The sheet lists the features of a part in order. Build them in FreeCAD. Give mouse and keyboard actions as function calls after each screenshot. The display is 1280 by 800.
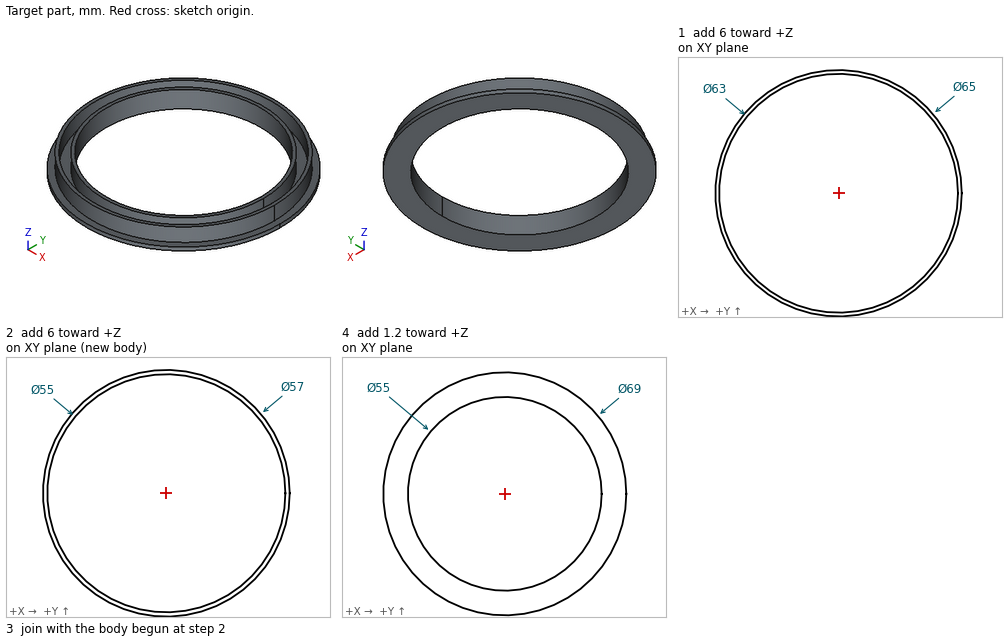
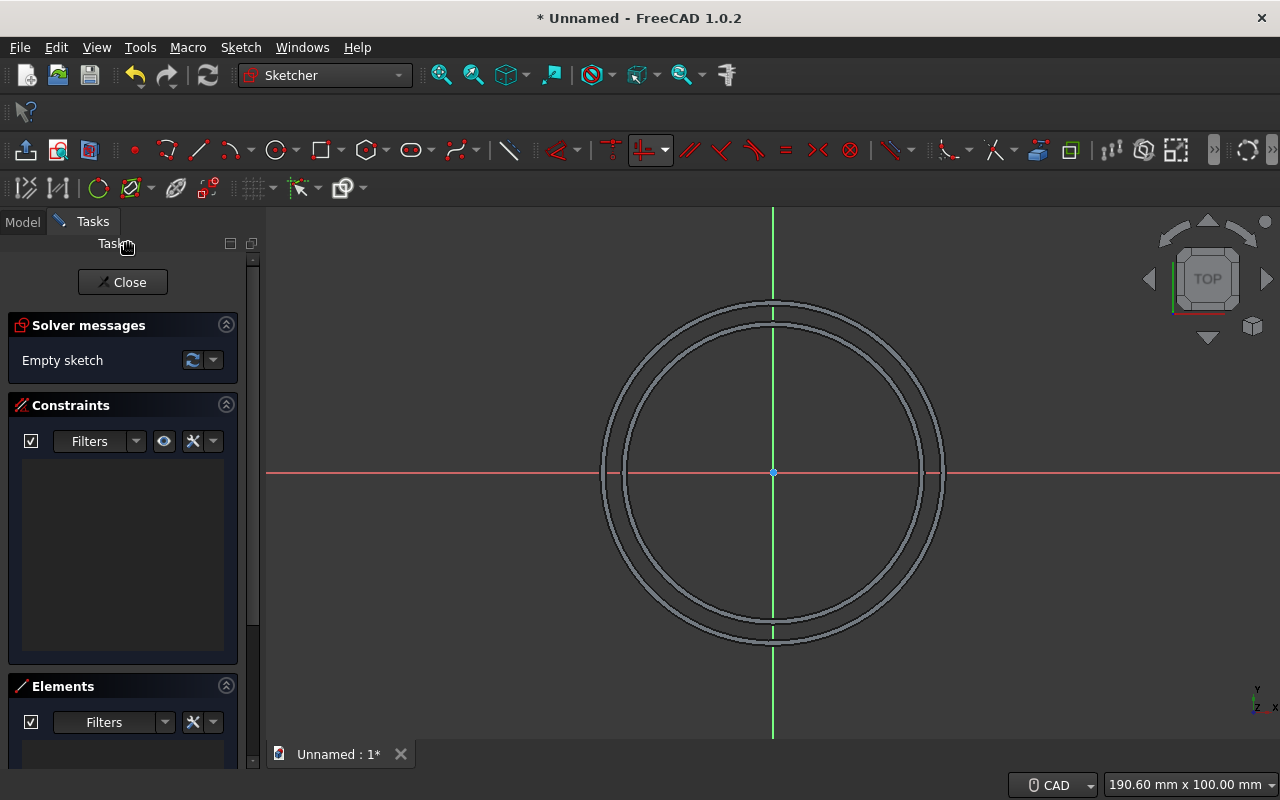
click(90, 150)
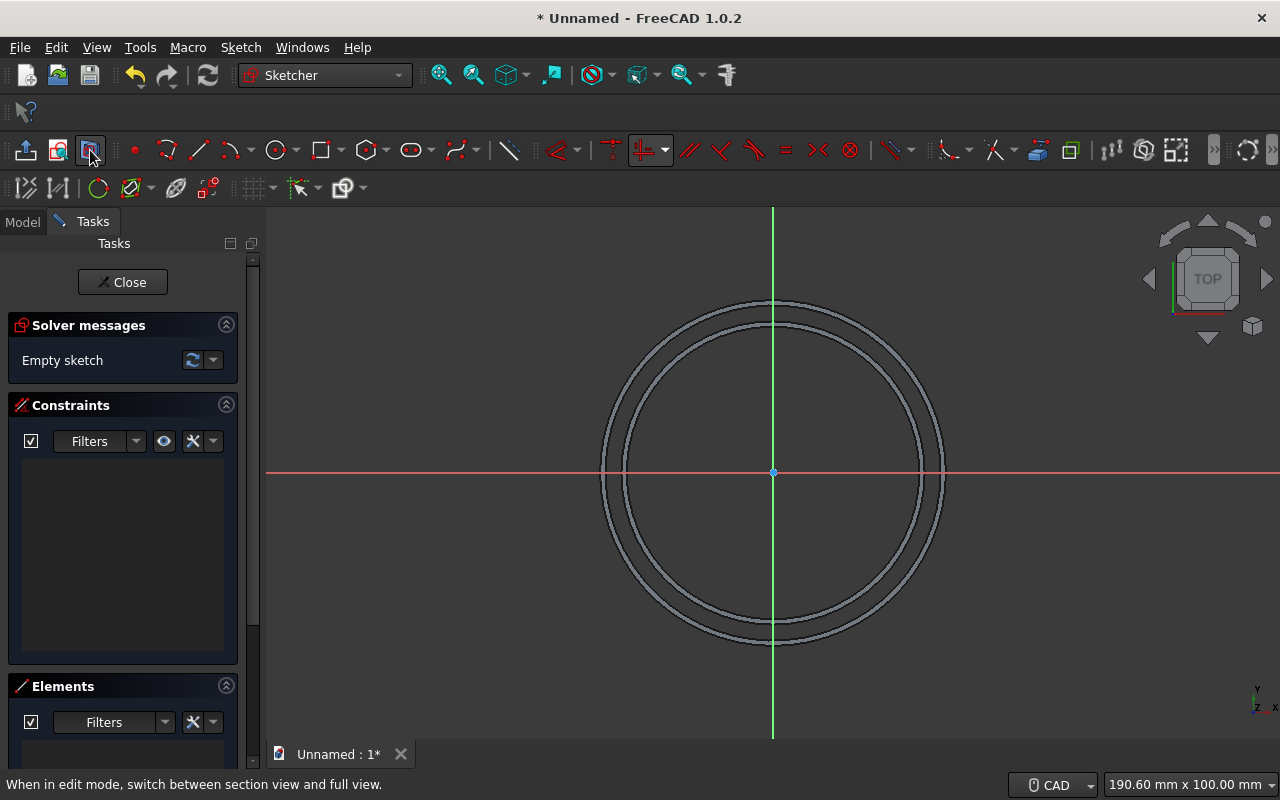
click(276, 150)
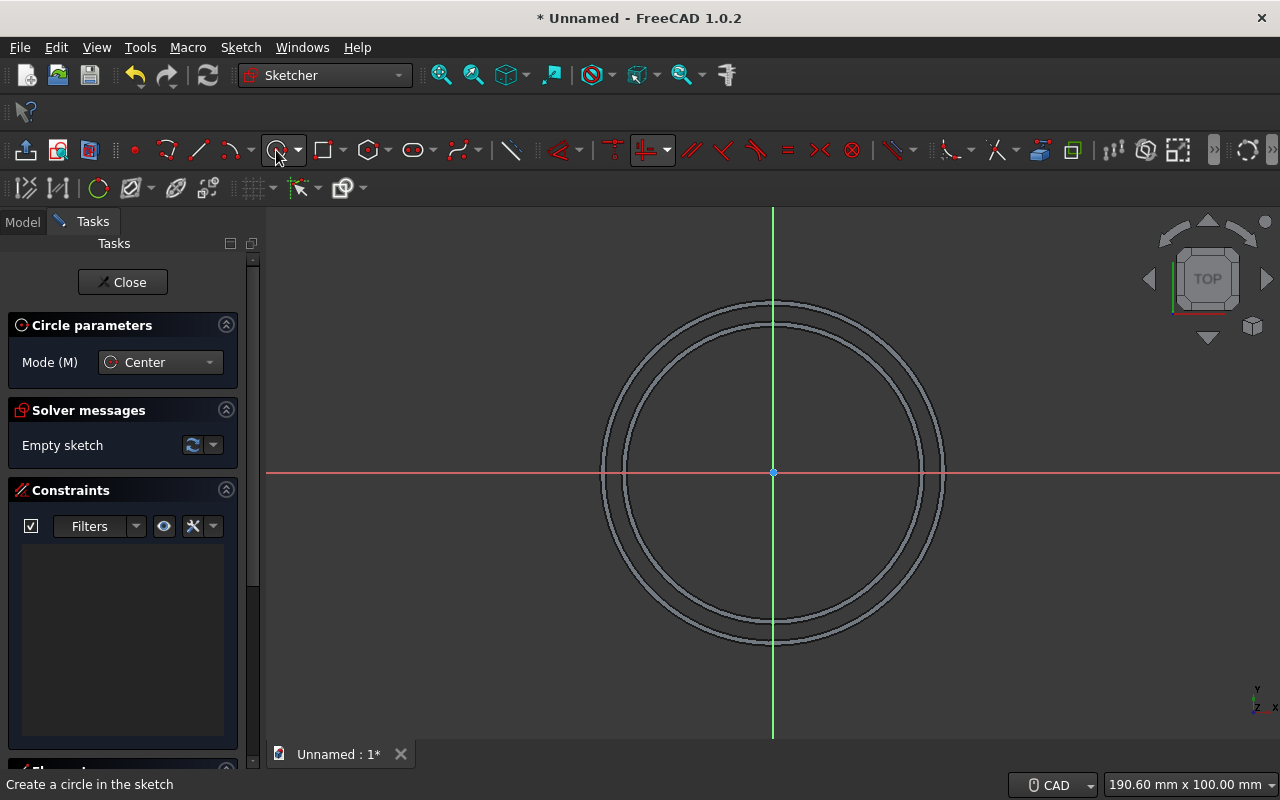
click(773, 473)
move(903, 343)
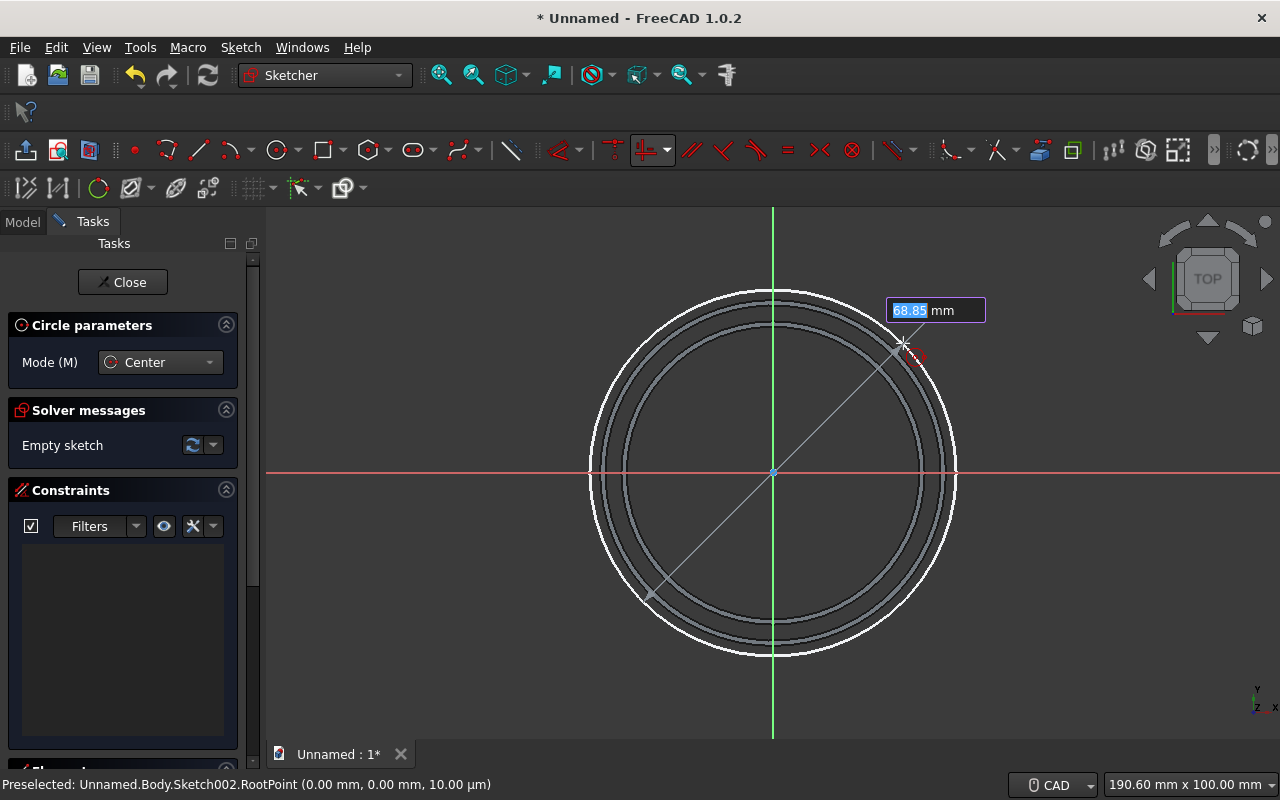
text(69)
key(Return)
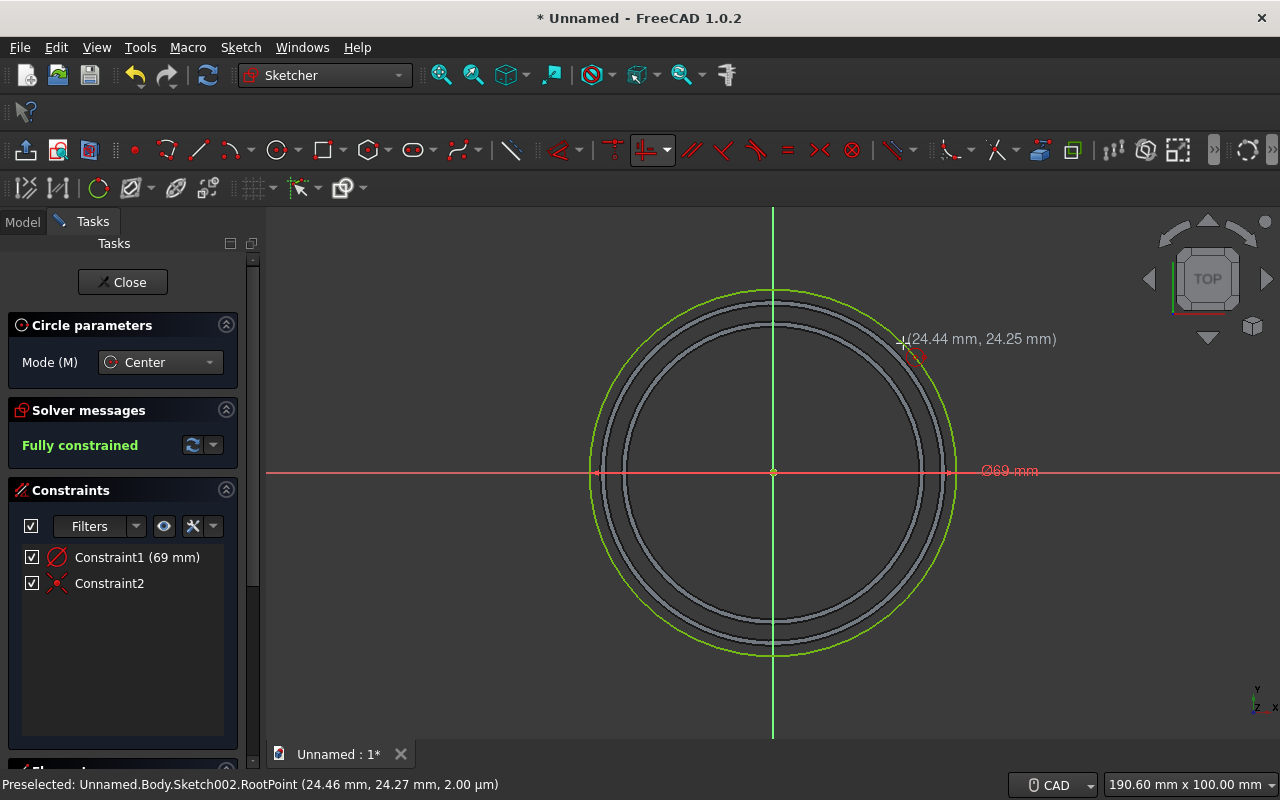
click(773, 473)
move(876, 370)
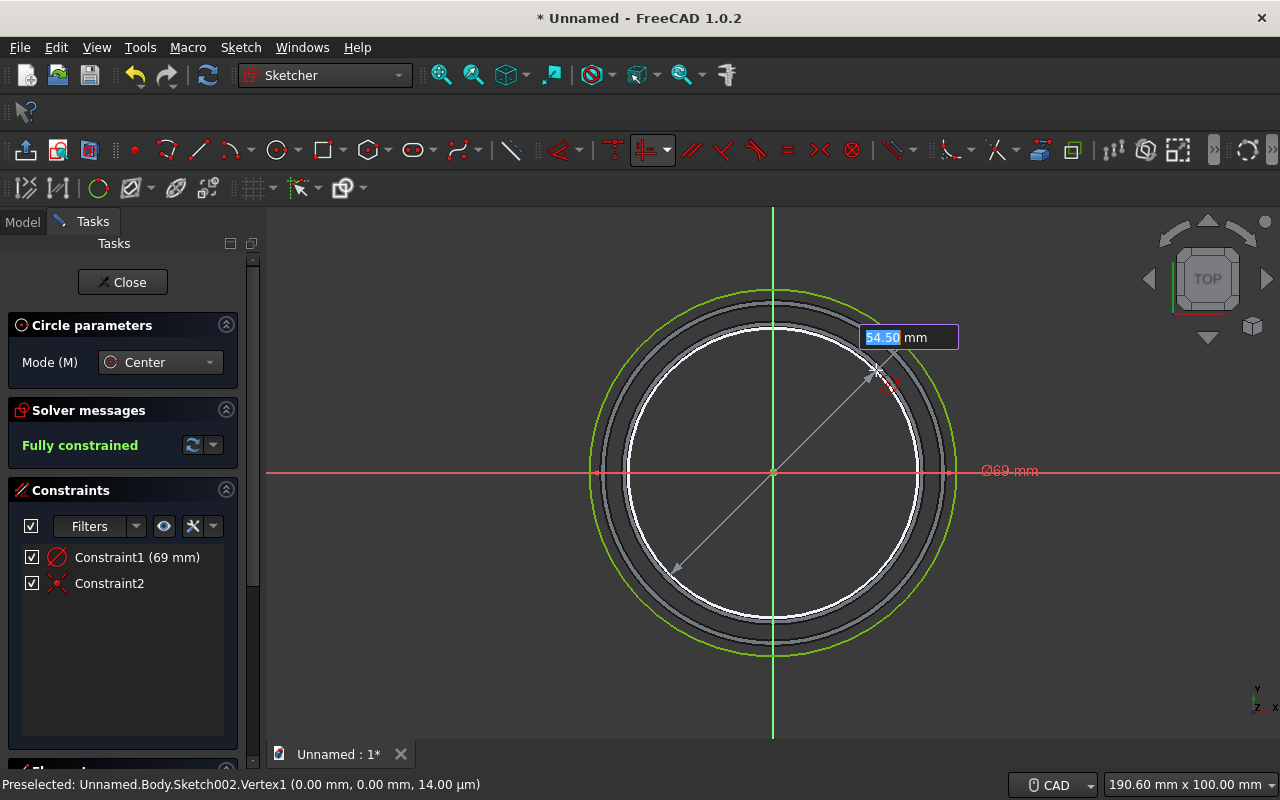
text(55)
key(Return)
key(Escape)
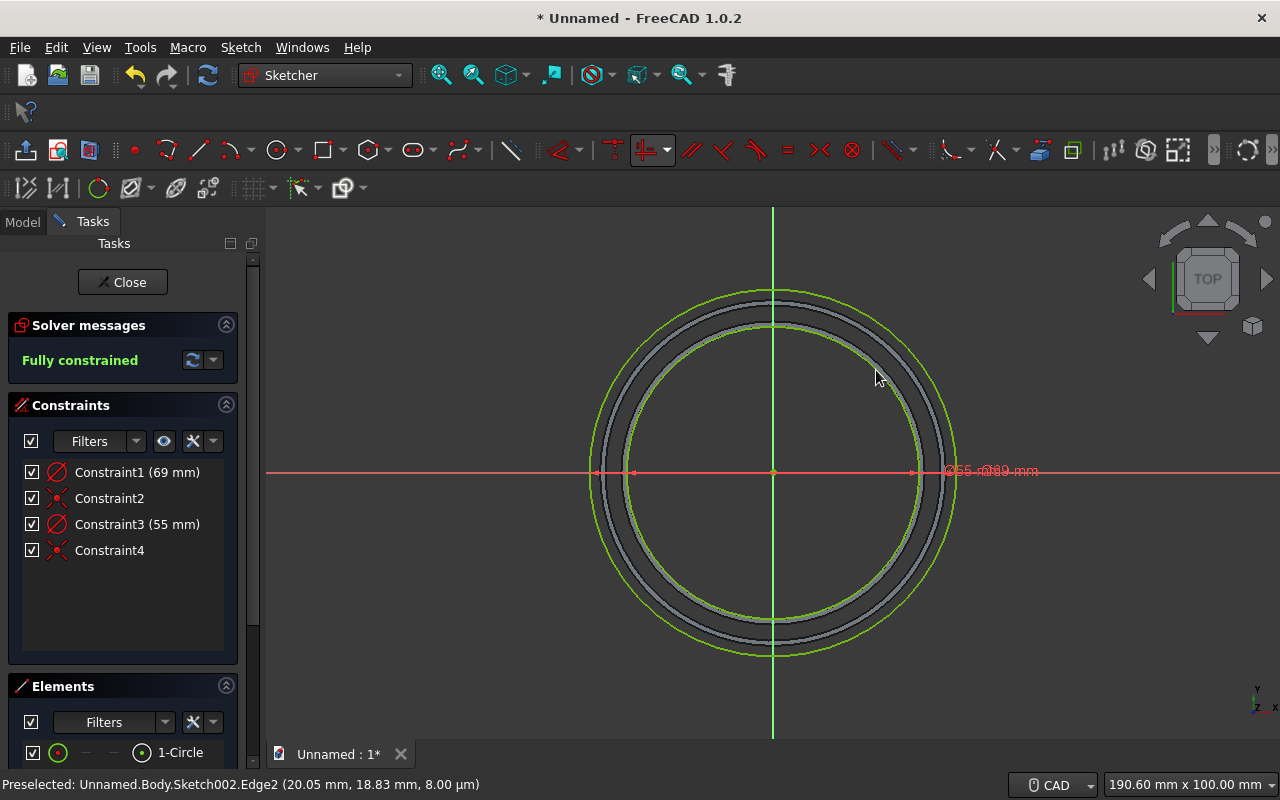
click(123, 282)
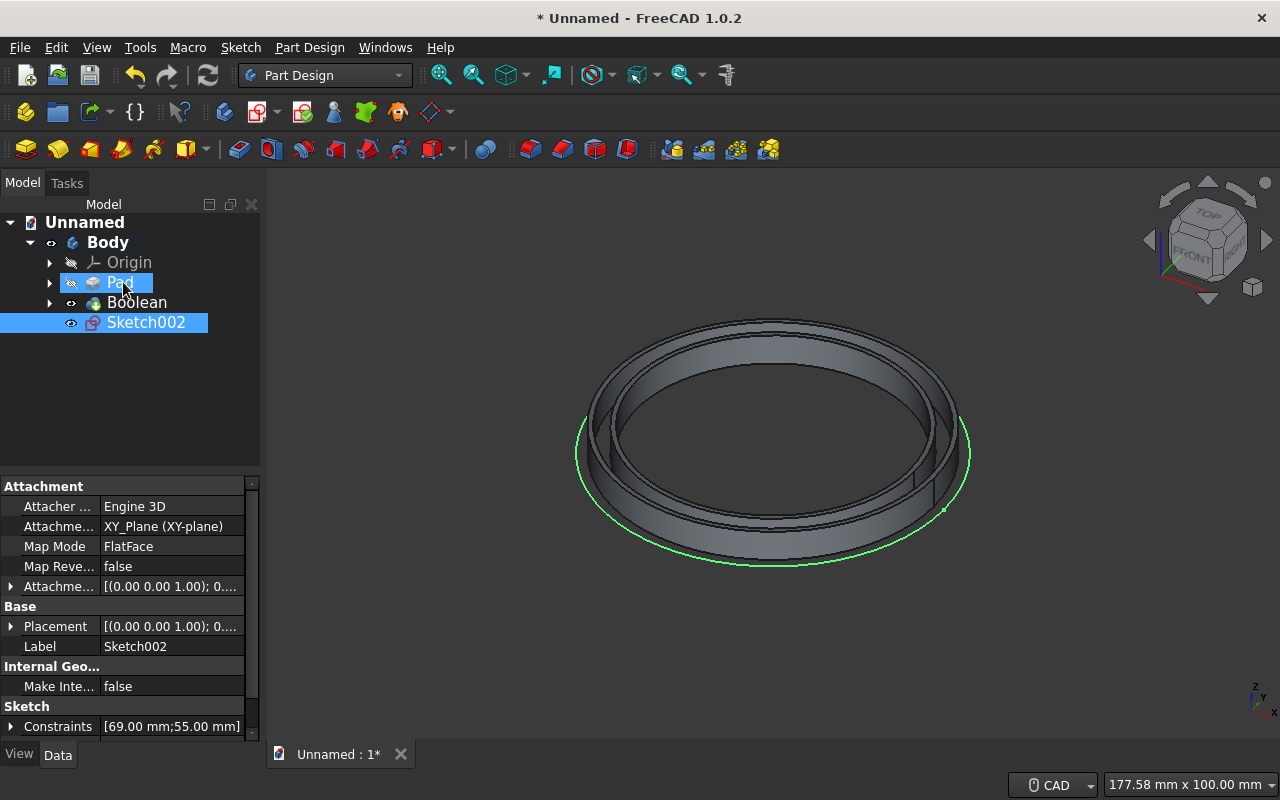
click(26, 150)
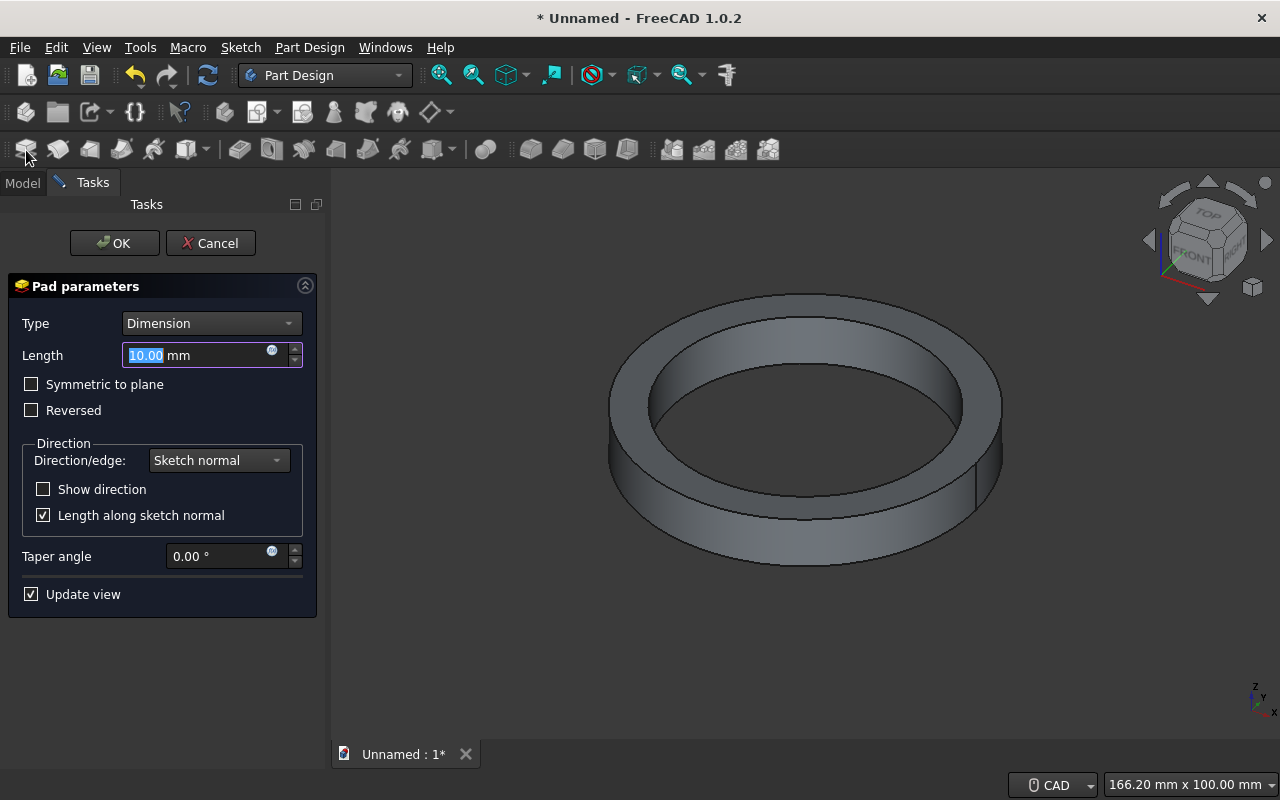
text(1.2)
key(Tab)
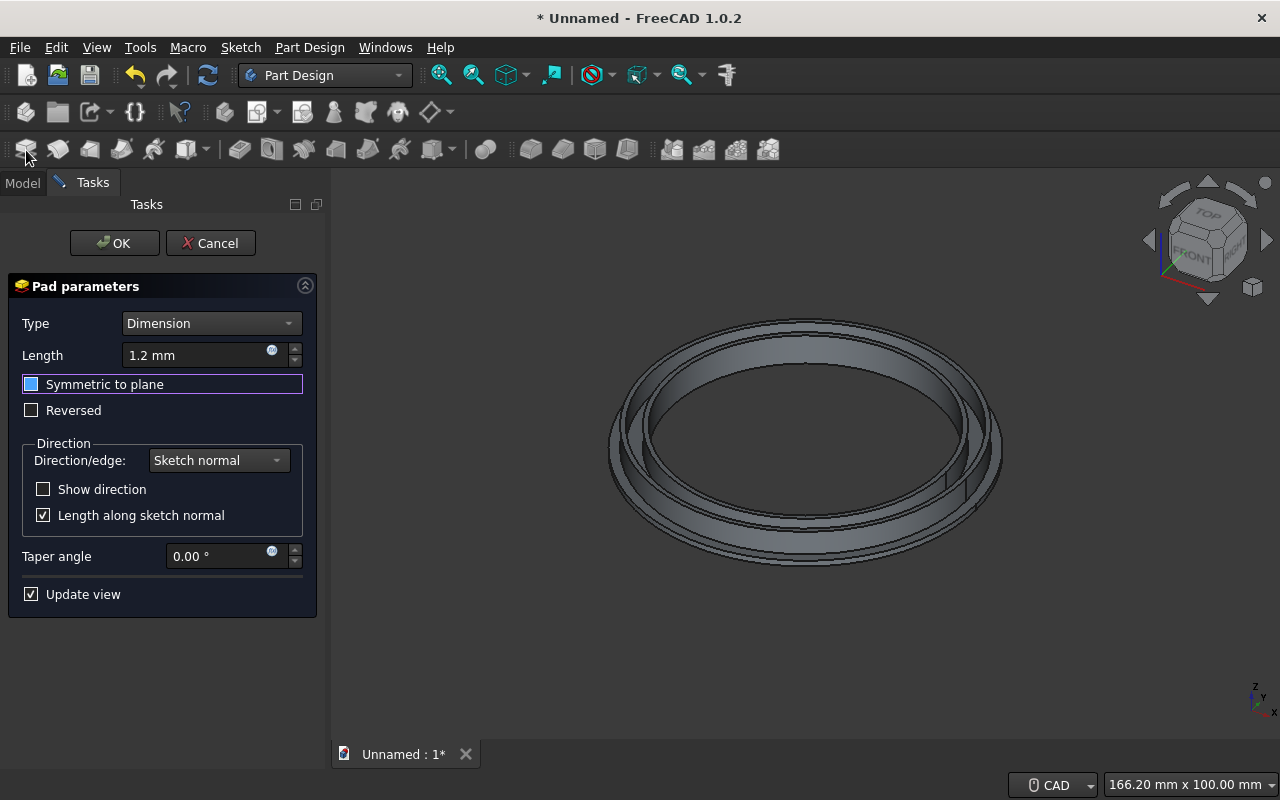
click(115, 243)